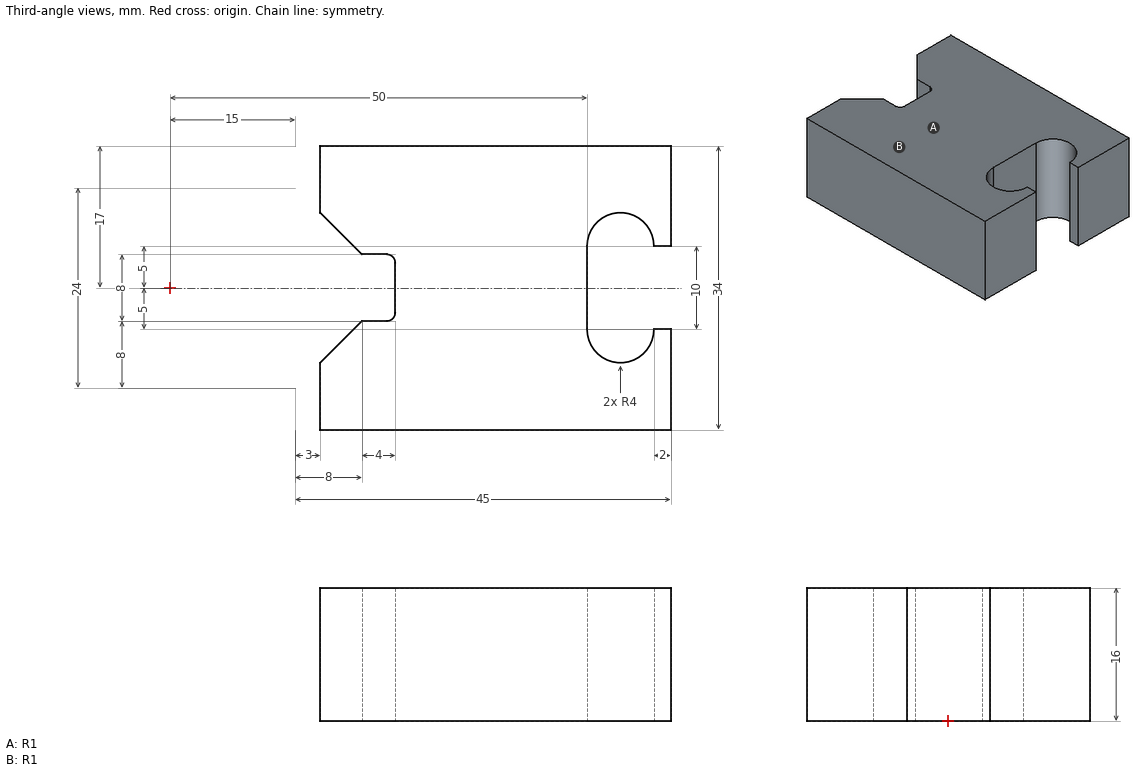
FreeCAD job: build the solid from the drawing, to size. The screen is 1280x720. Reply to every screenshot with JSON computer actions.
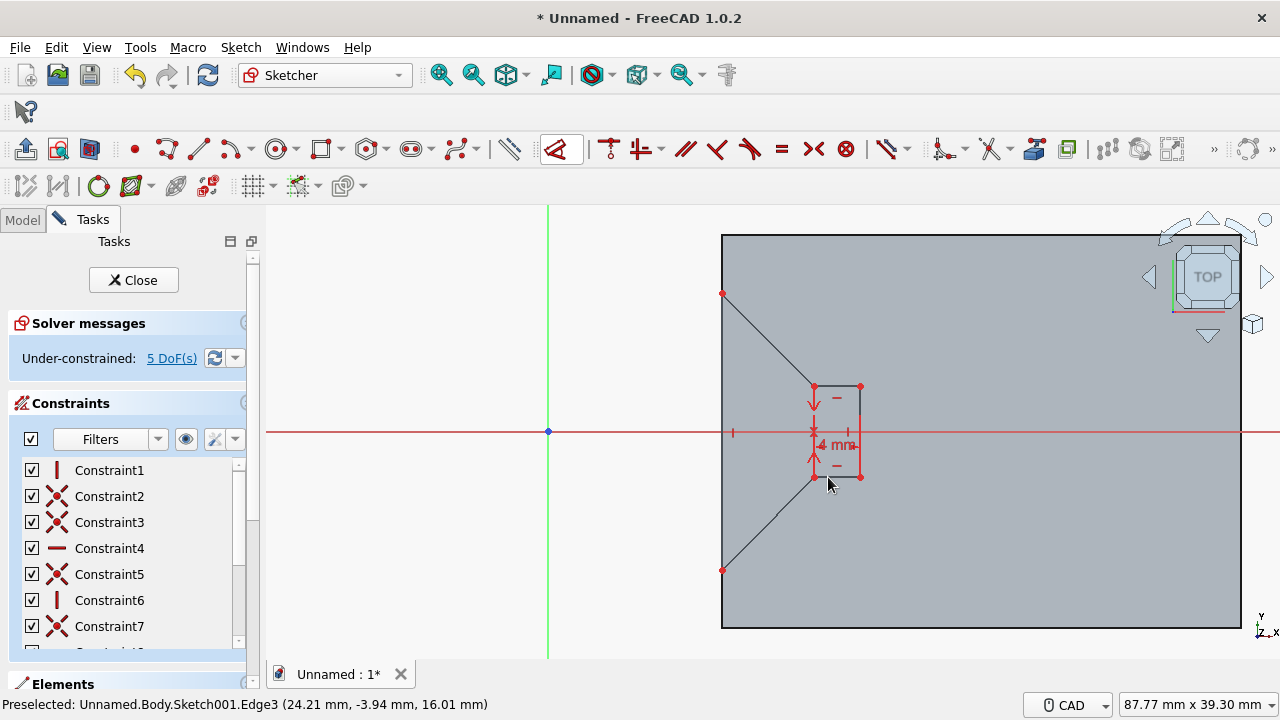
{"action": "left_click", "coordinate": [860, 450]}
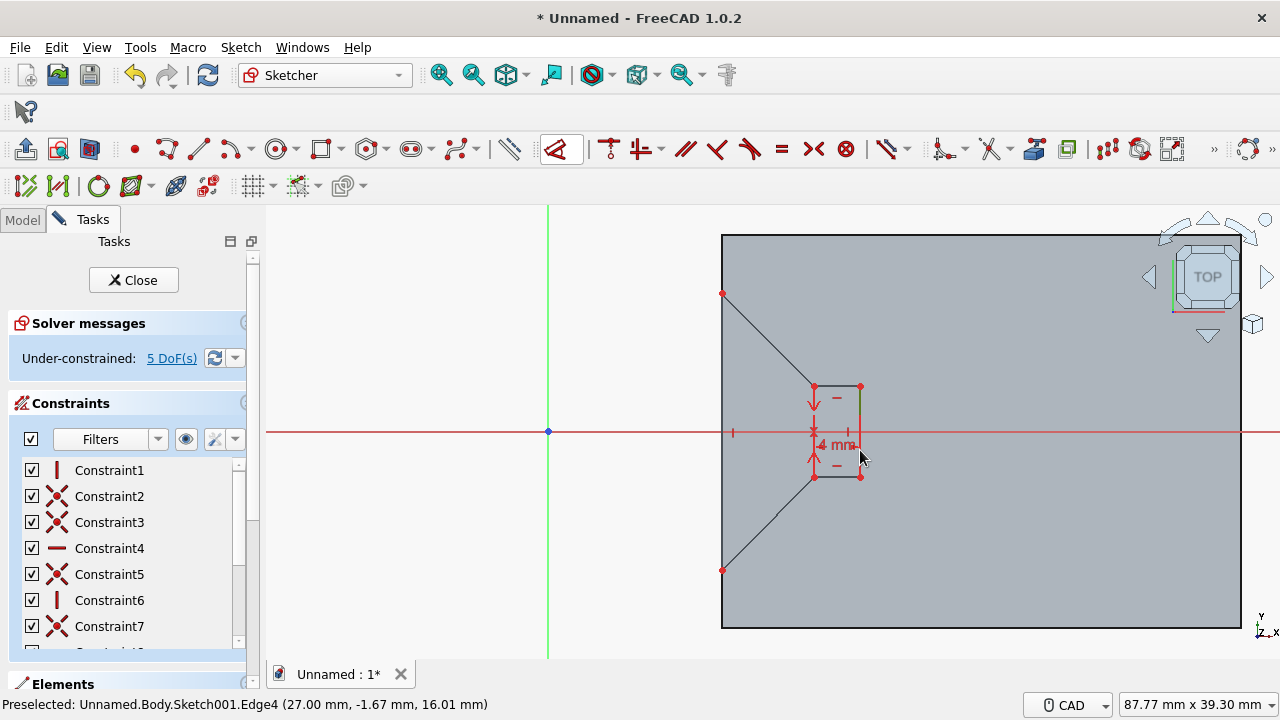
{"action": "left_click", "coordinate": [578, 150]}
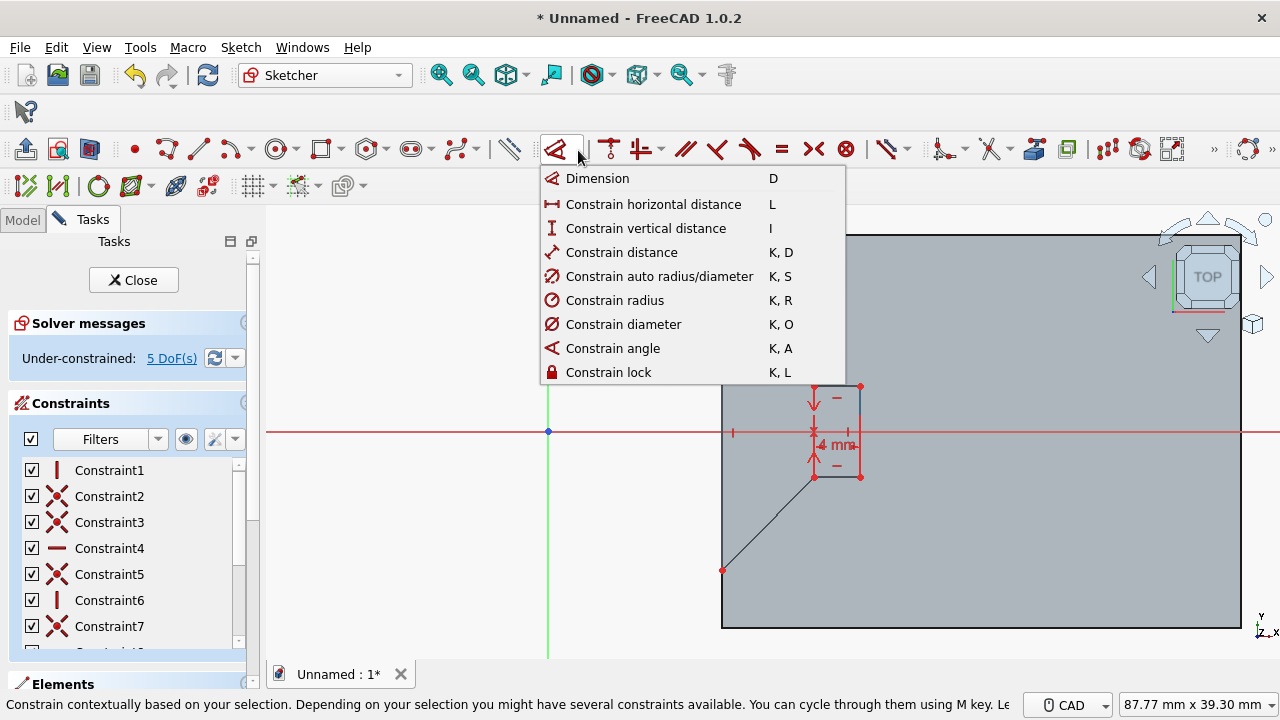
{"action": "left_click", "coordinate": [693, 228]}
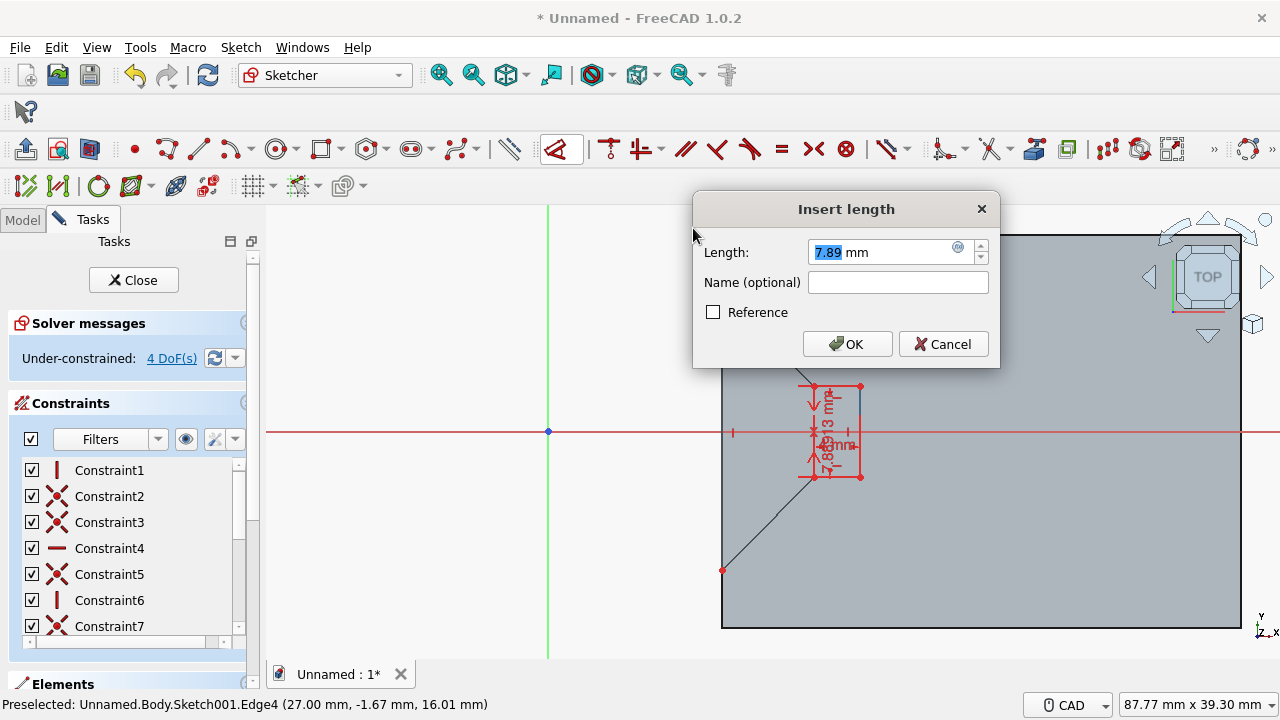
{"action": "type", "text": "8"}
{"action": "key", "text": "Return"}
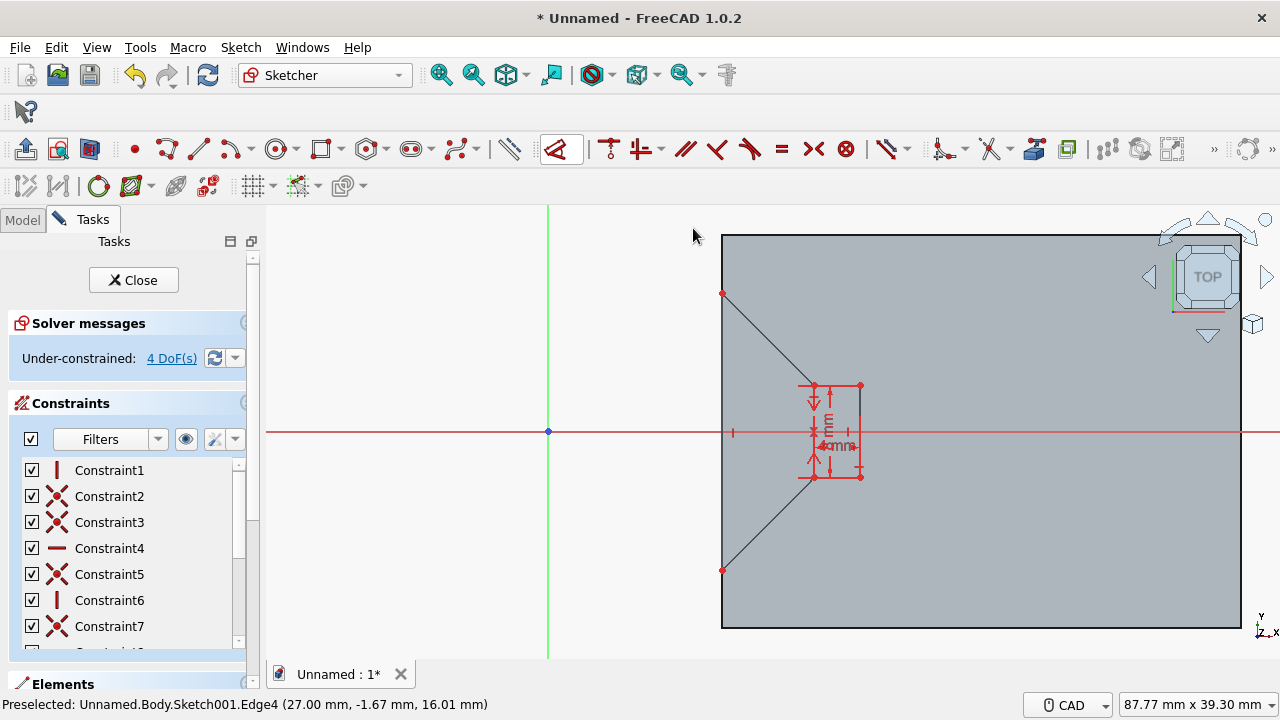
{"action": "left_click", "coordinate": [722, 377]}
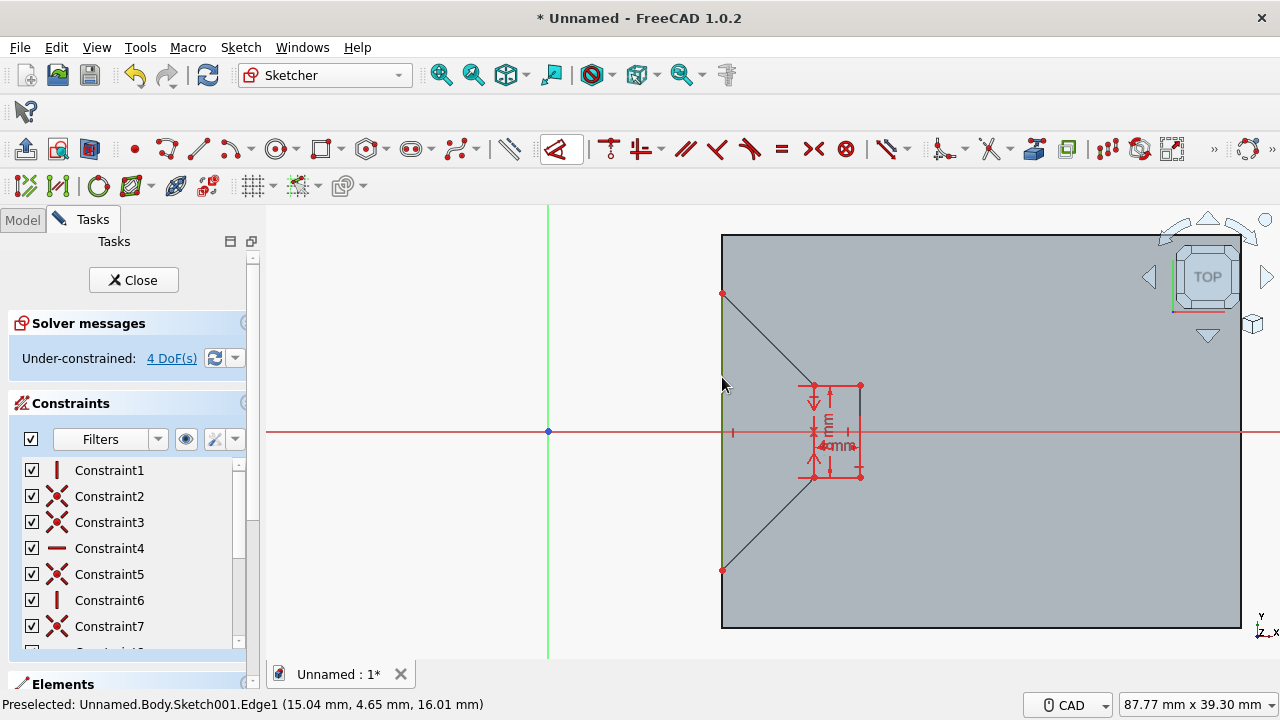
{"action": "left_click", "coordinate": [578, 150]}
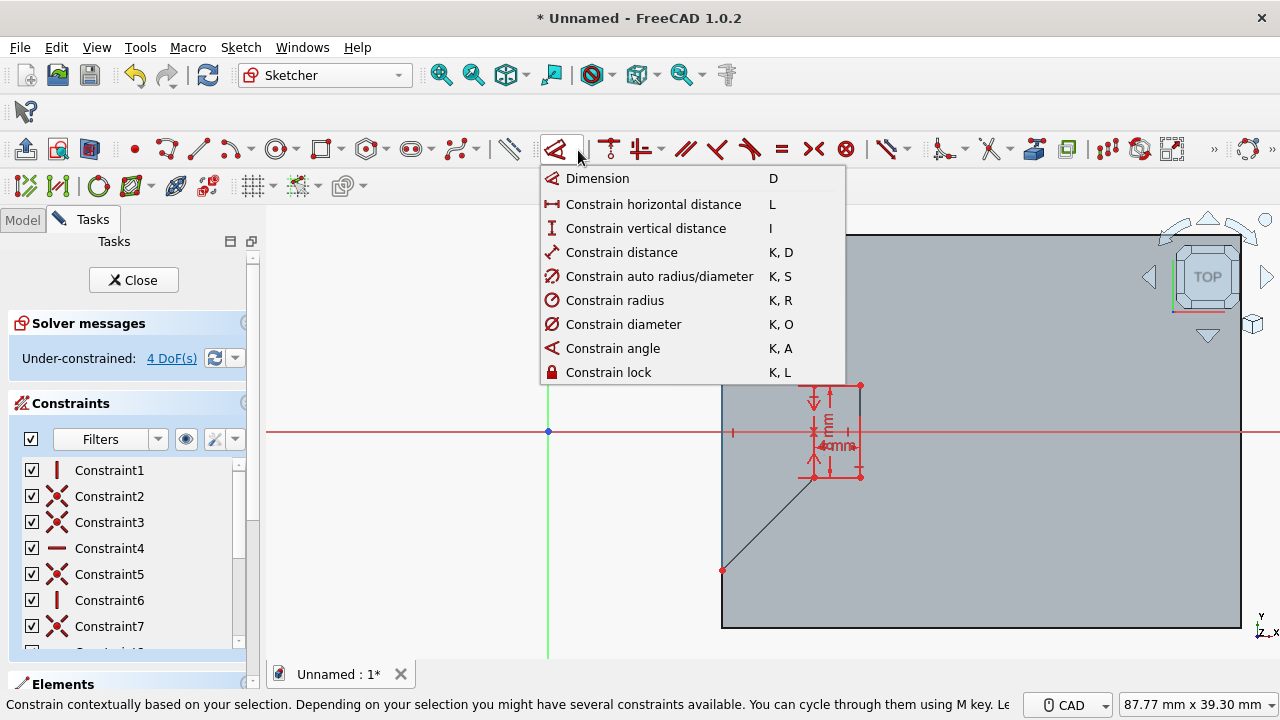
{"action": "left_click", "coordinate": [693, 228]}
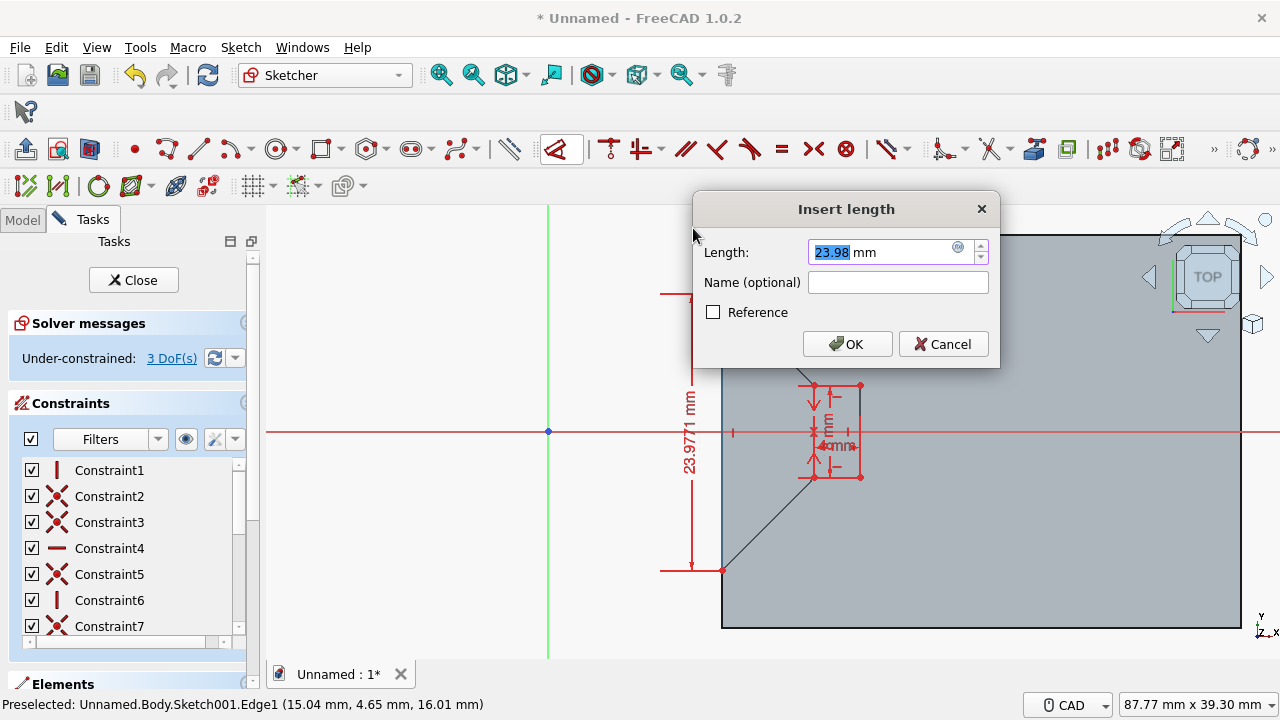
{"action": "type", "text": "24"}
{"action": "key", "text": "Return"}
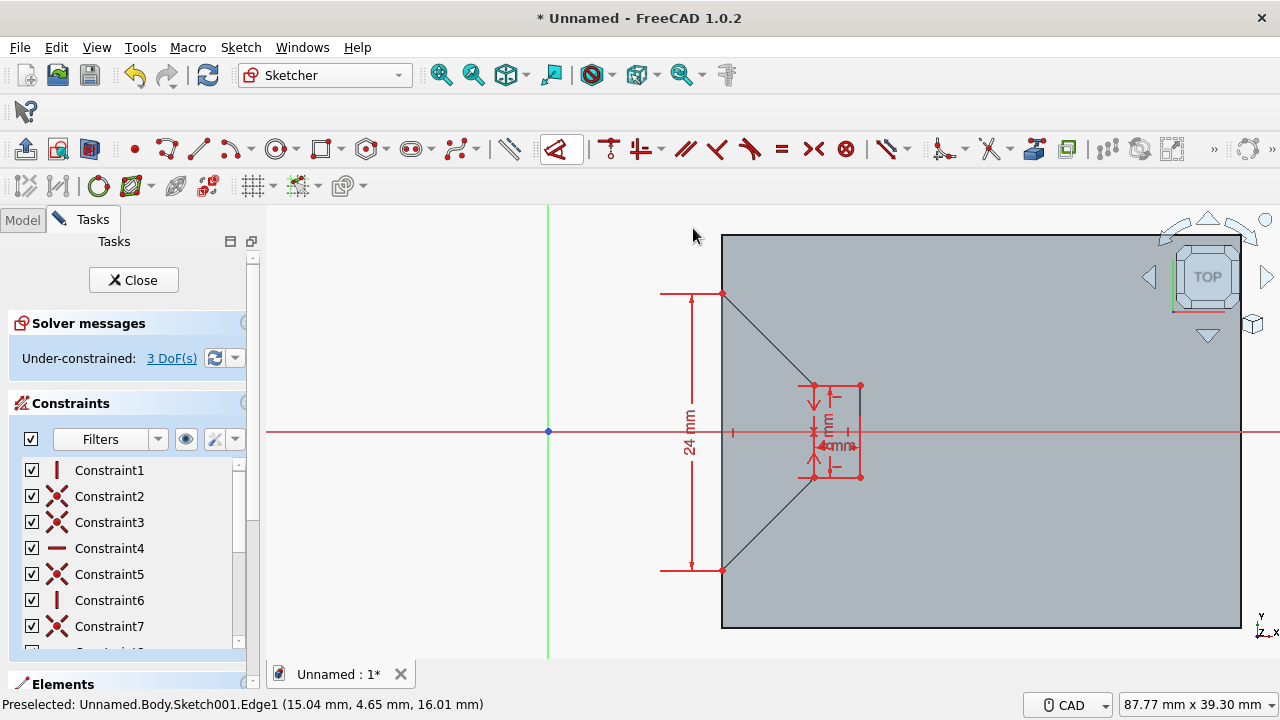
{"action": "left_click", "coordinate": [750, 543]}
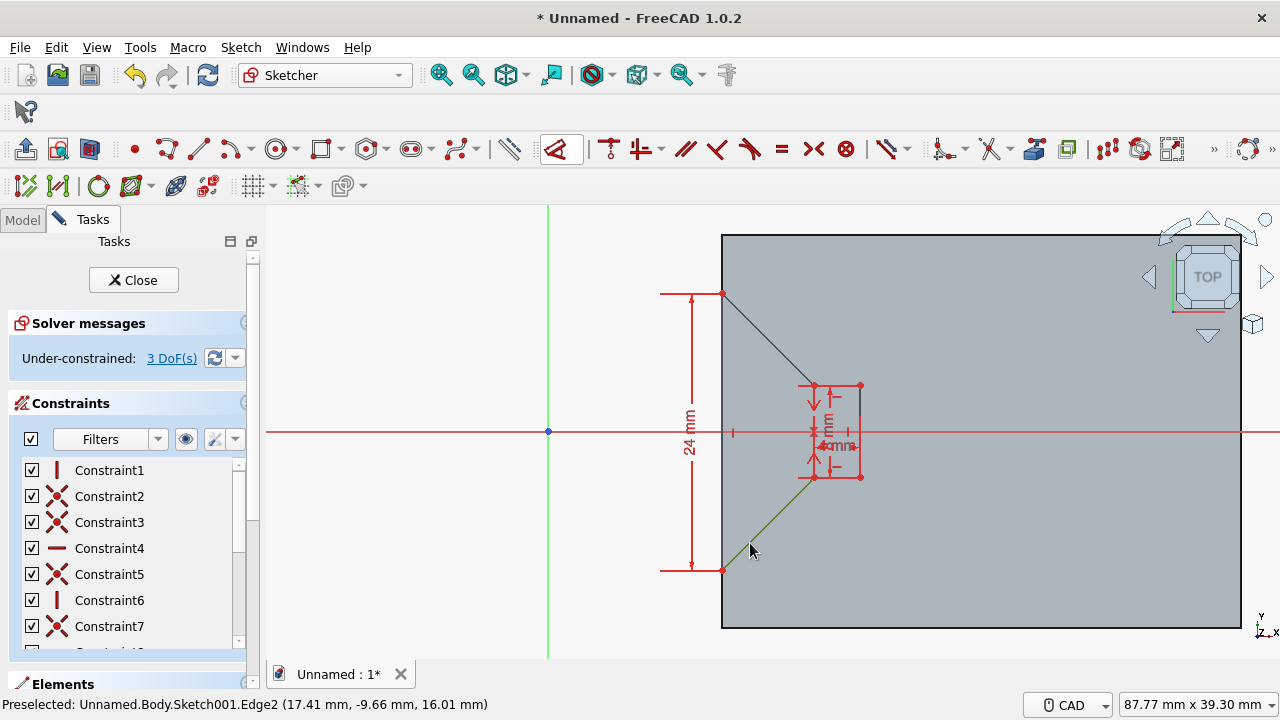
{"action": "key", "text": "l"}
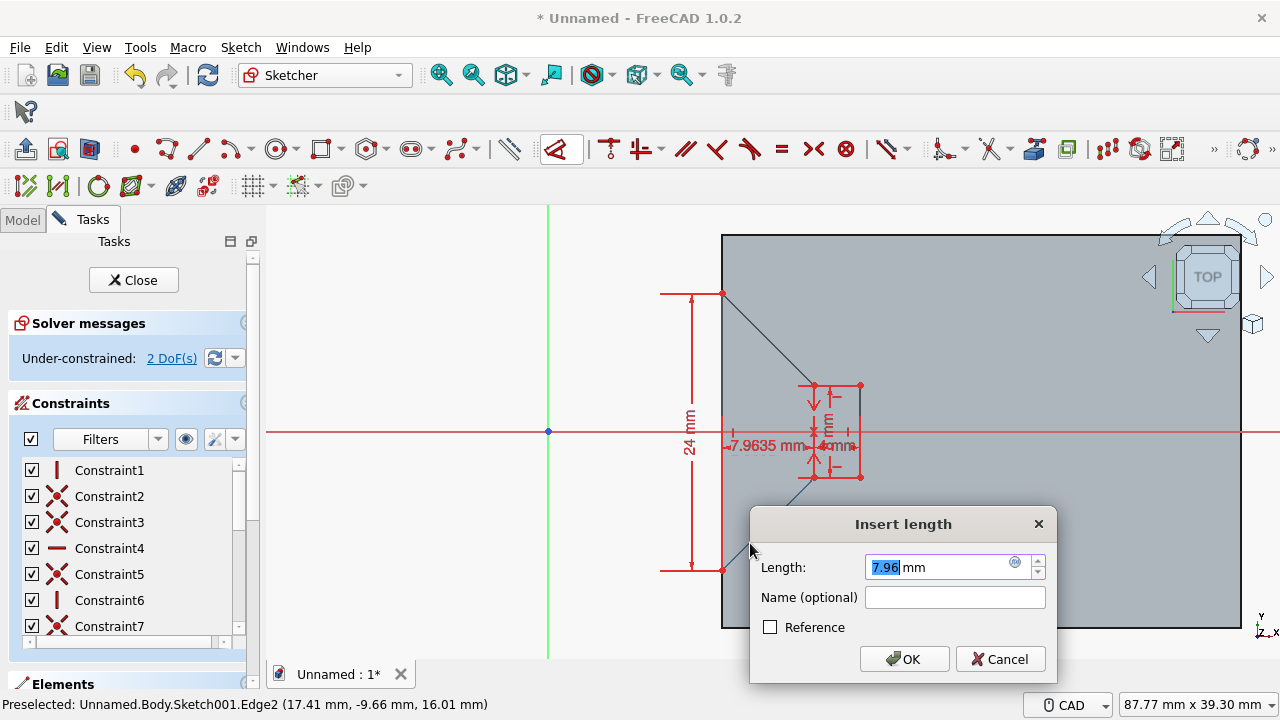
{"action": "type", "text": "8"}
{"action": "key", "text": "Return"}